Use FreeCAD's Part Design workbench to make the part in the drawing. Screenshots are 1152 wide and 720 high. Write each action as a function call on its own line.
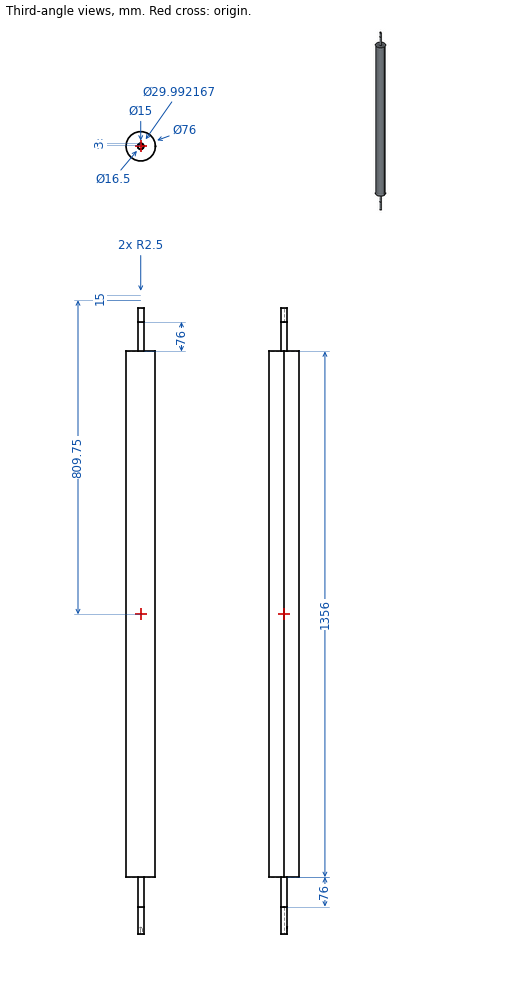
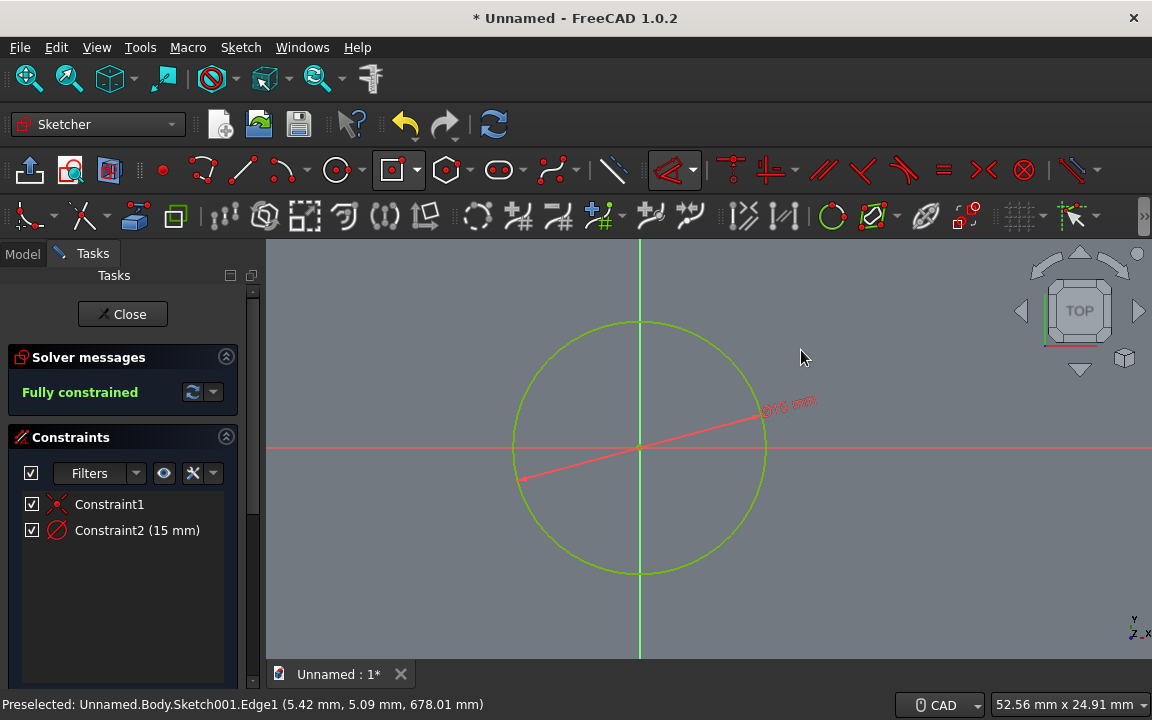
click(123, 314)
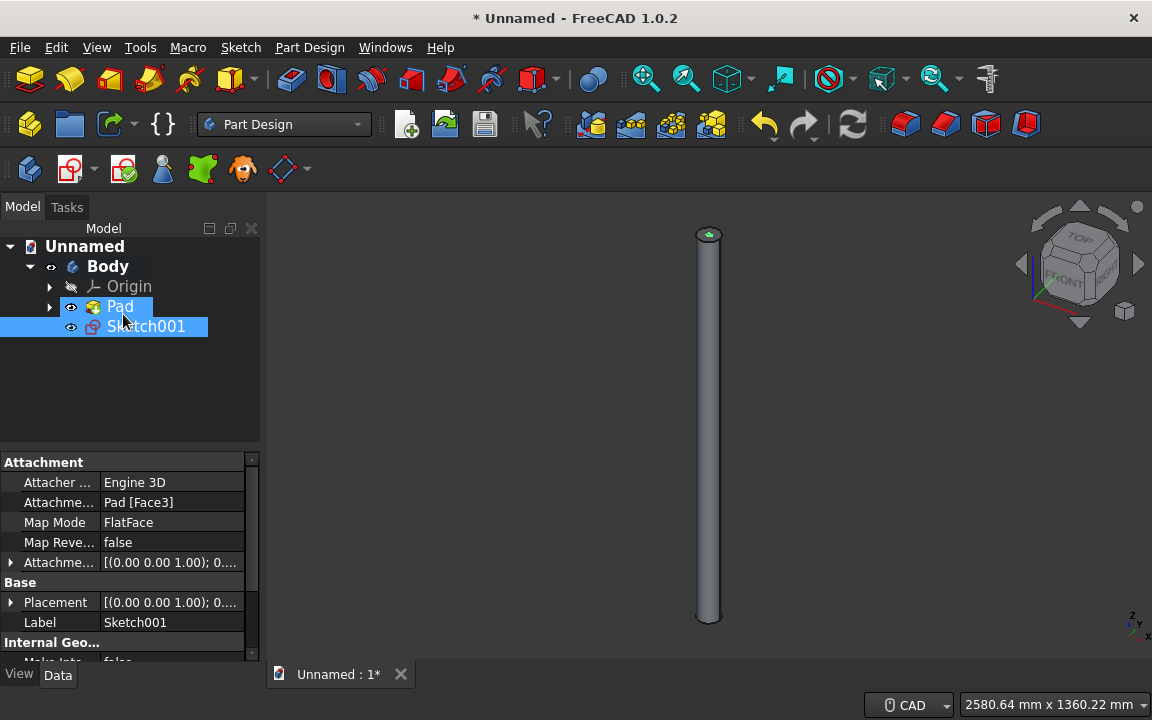
click(30, 80)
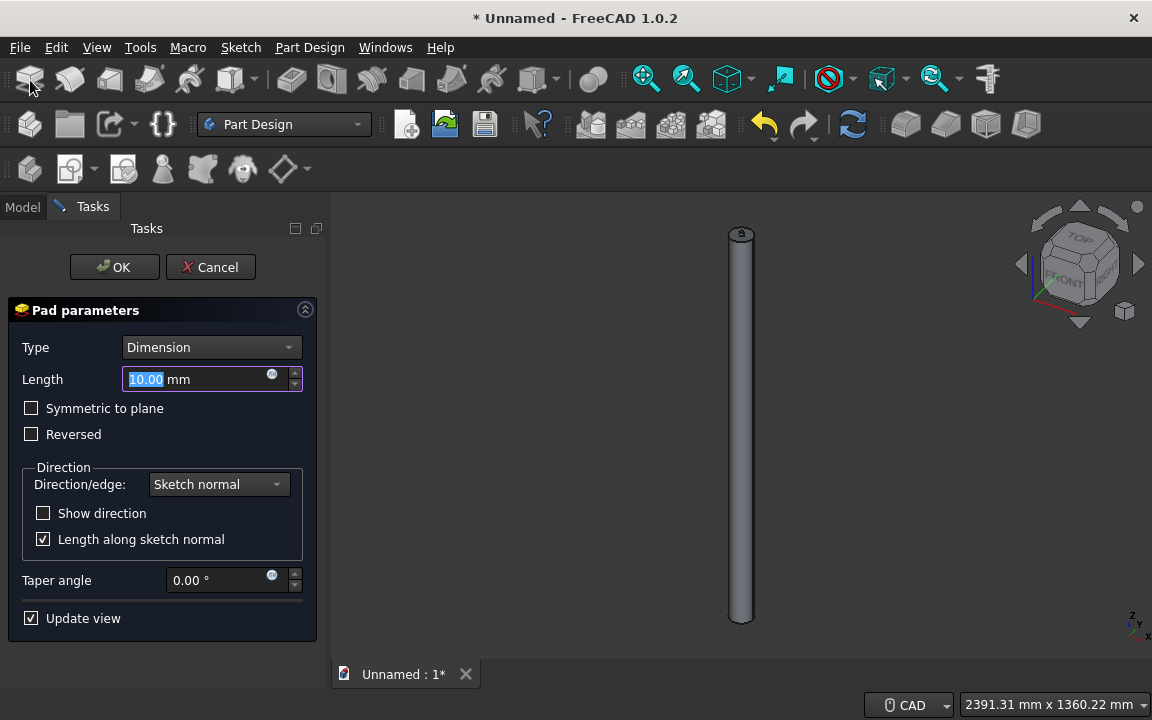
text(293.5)
key(Tab)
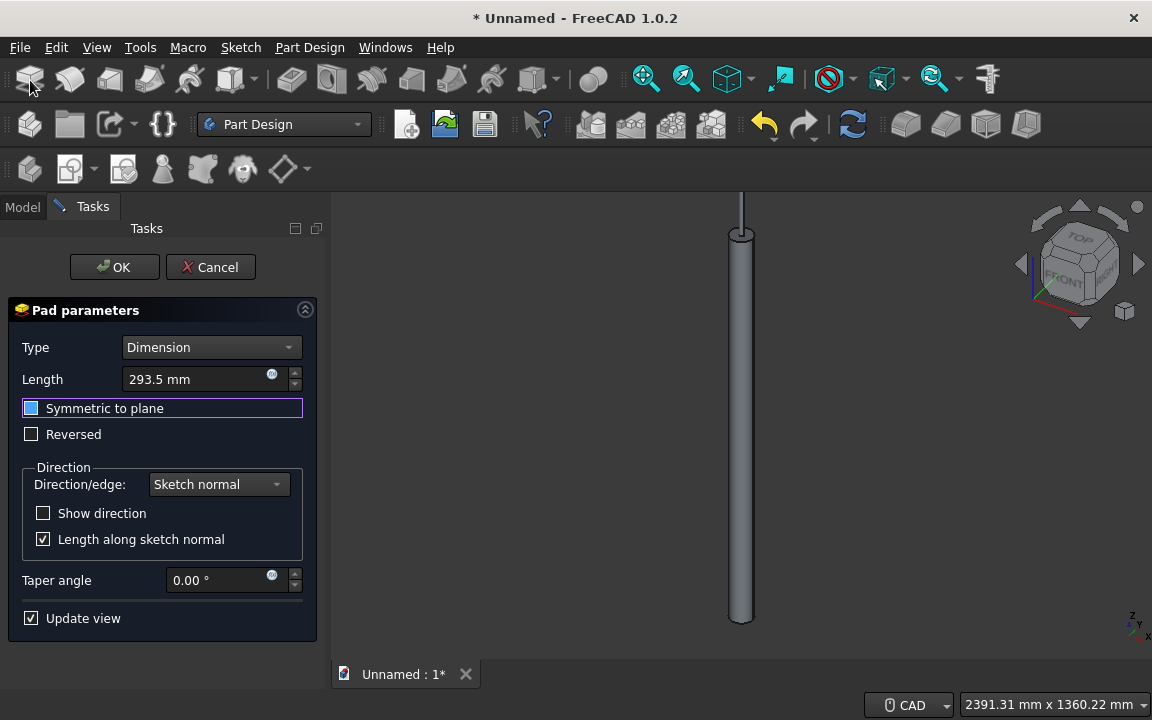
click(30, 408)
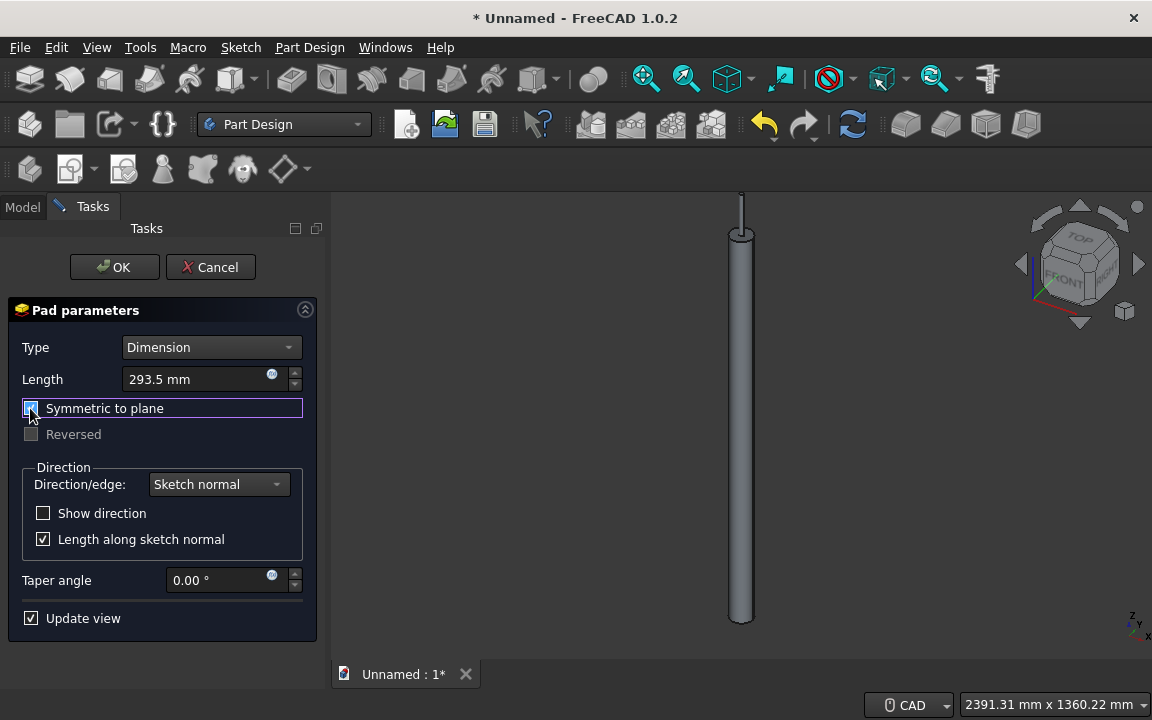
click(115, 267)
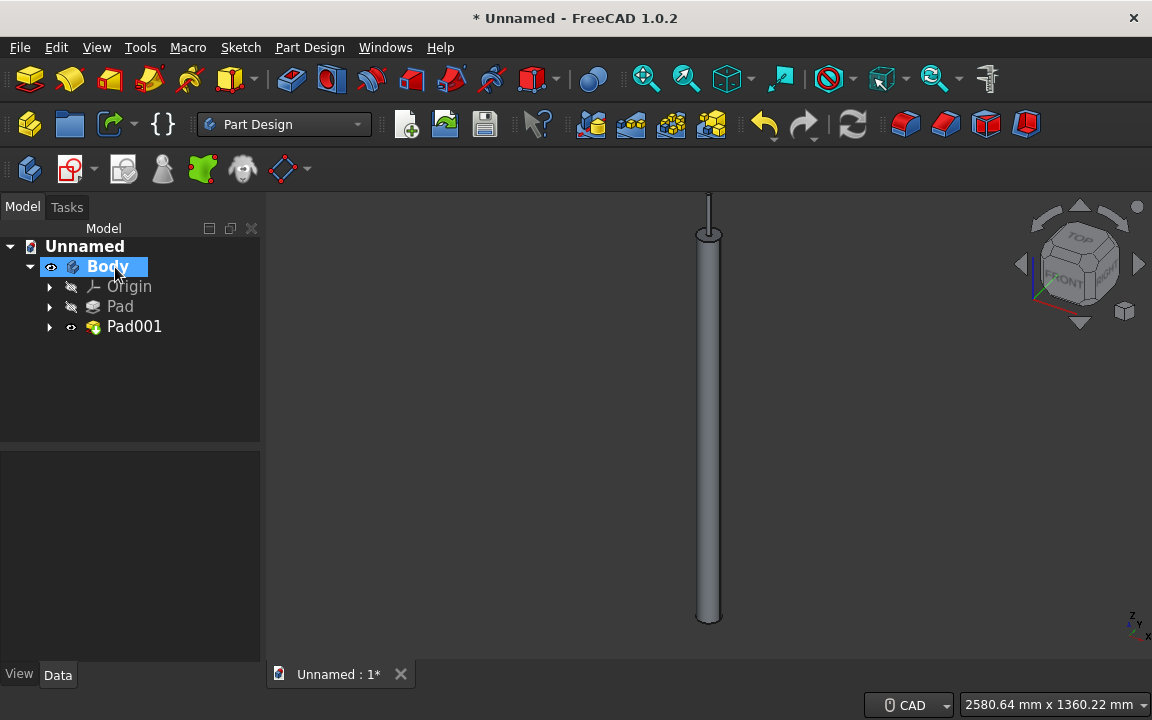
click(648, 80)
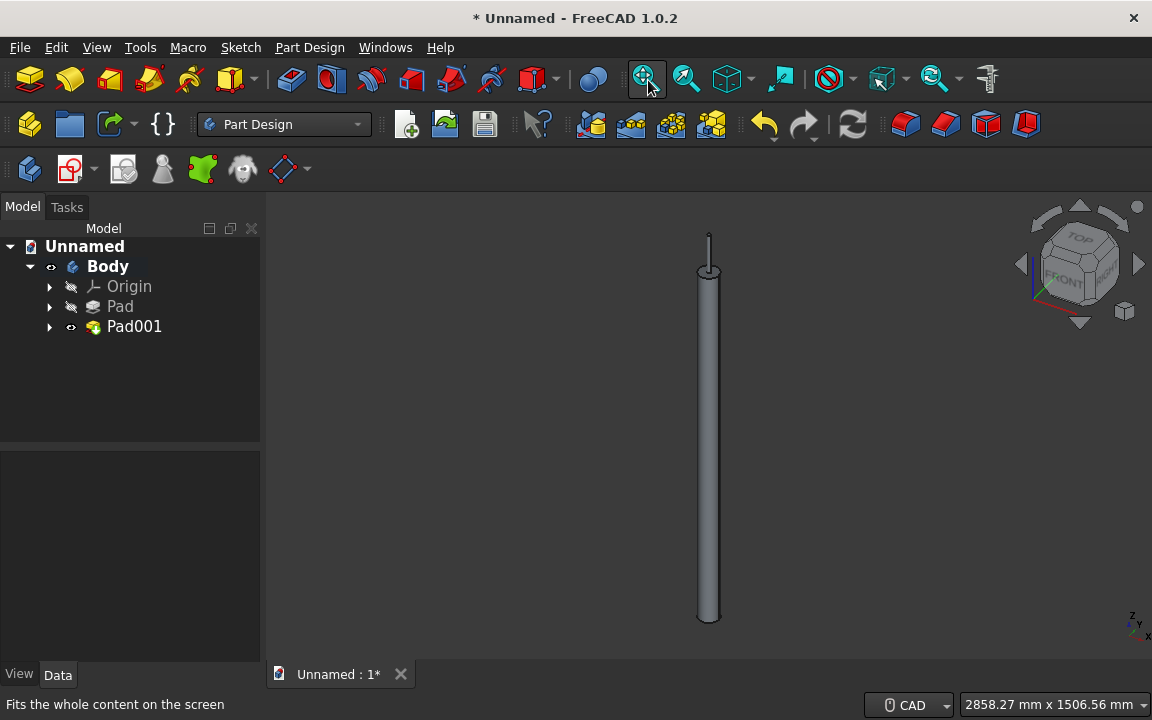
click(116, 327)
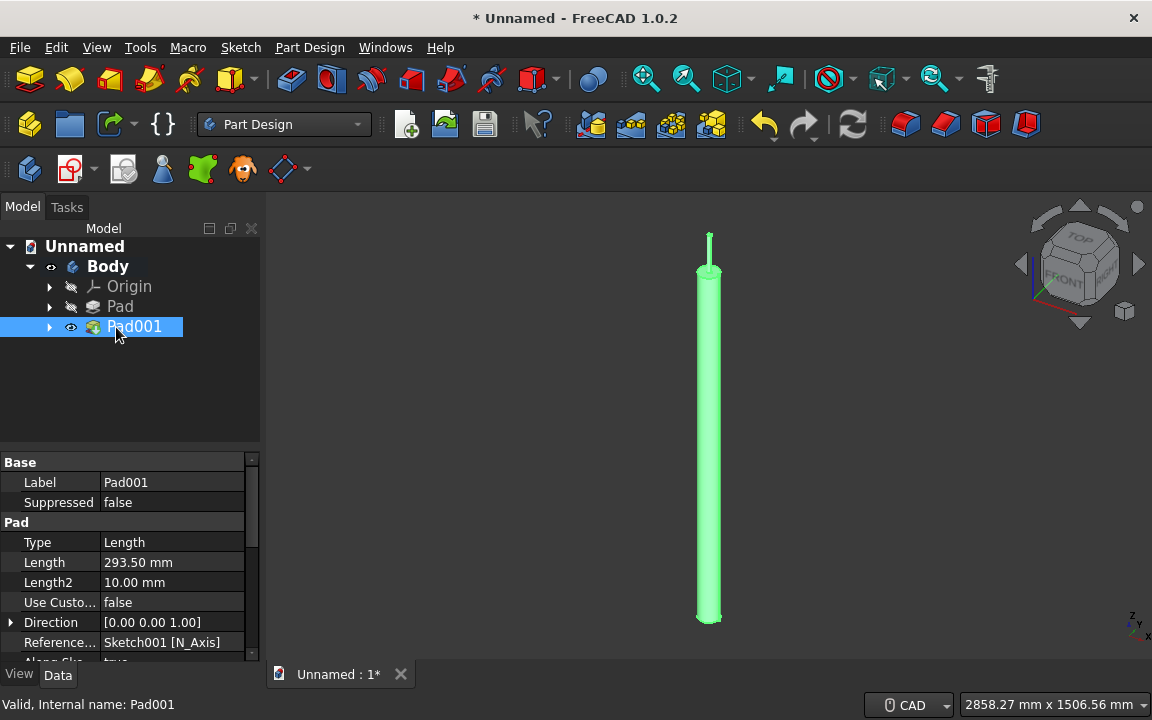
click(592, 124)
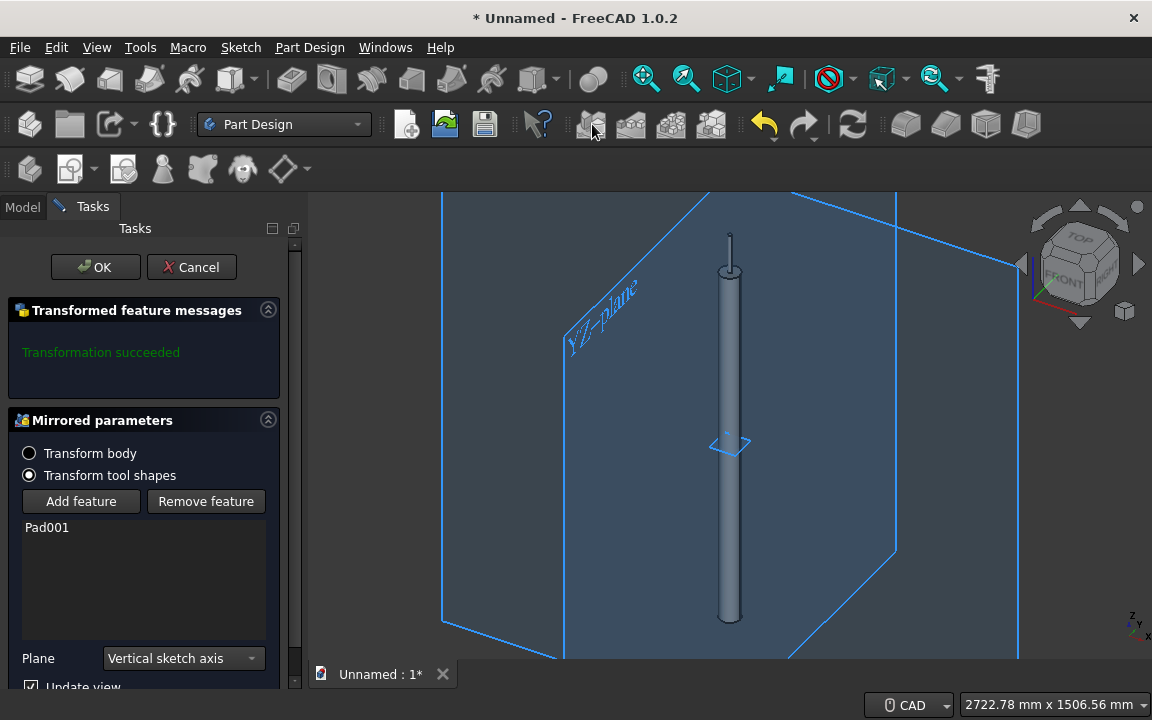
click(184, 658)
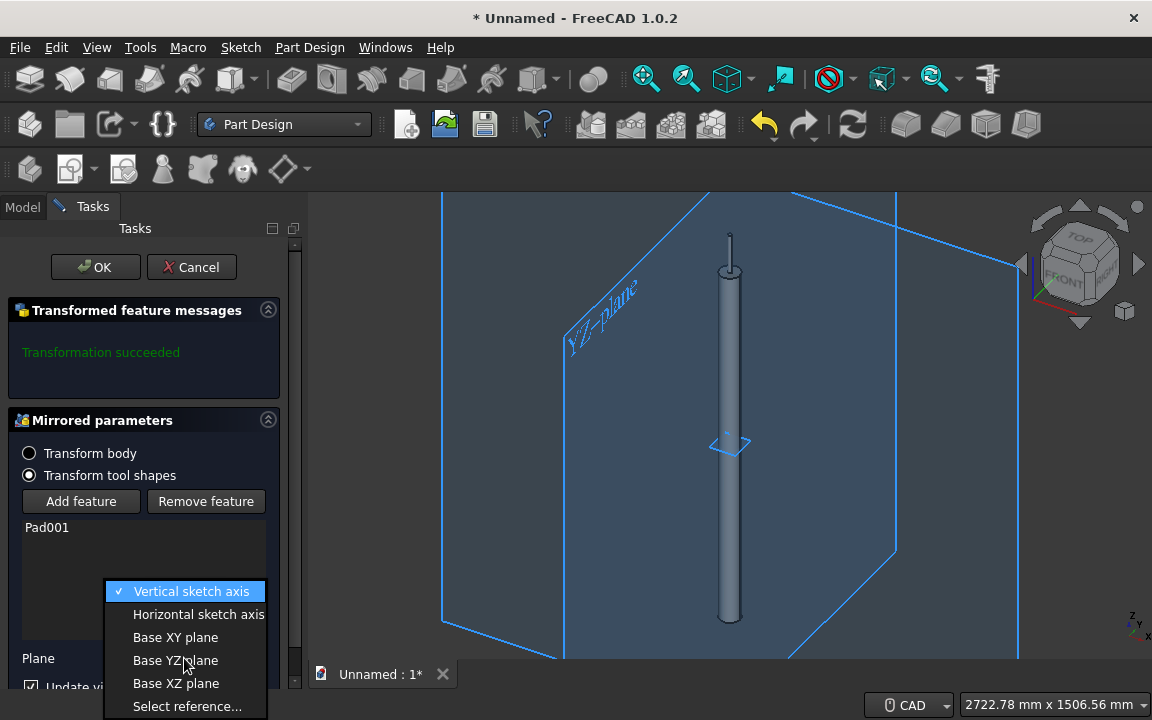
click(184, 638)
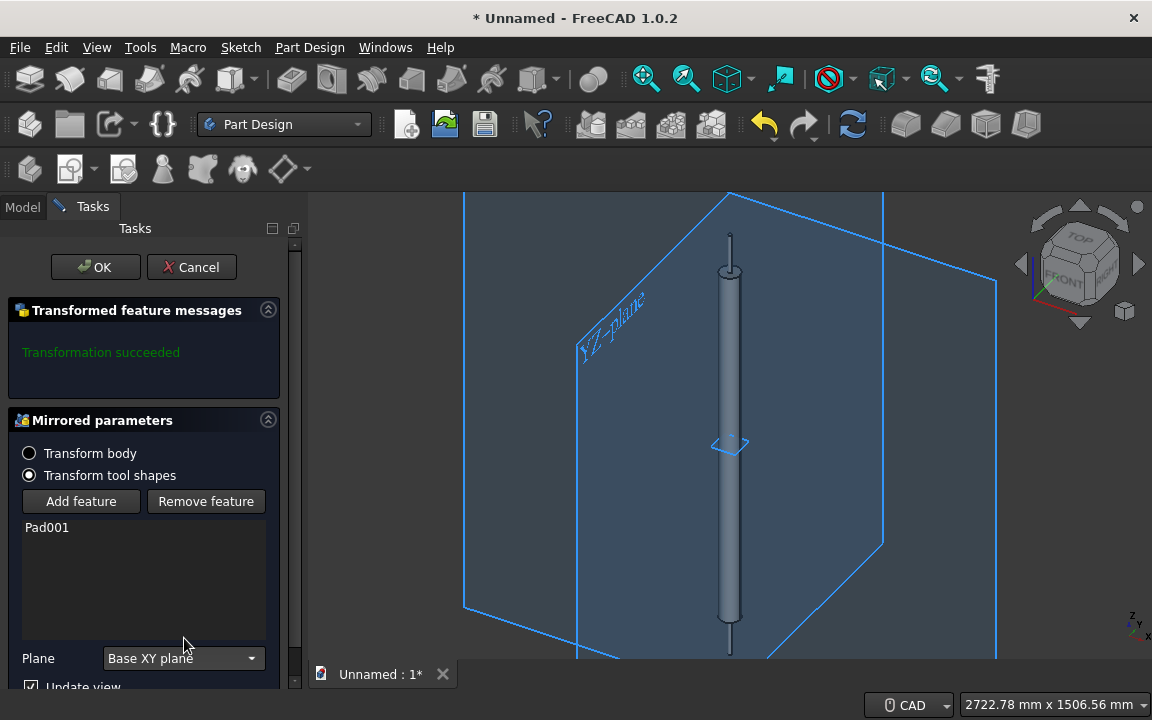
click(96, 267)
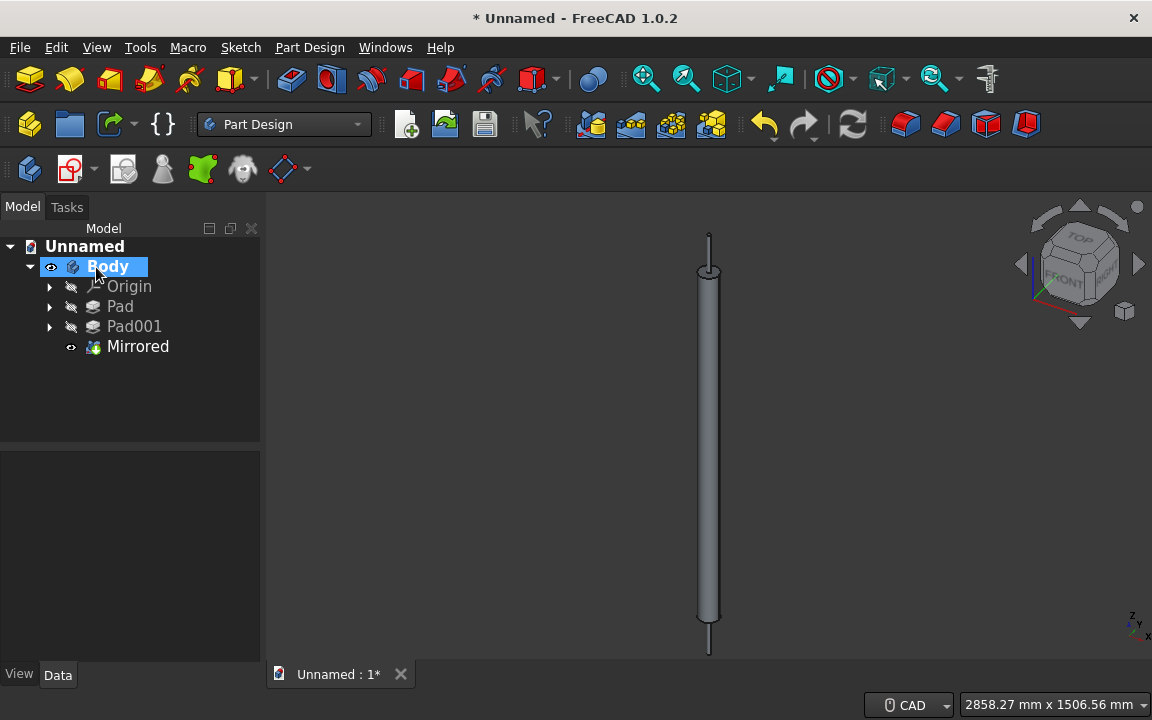
click(648, 80)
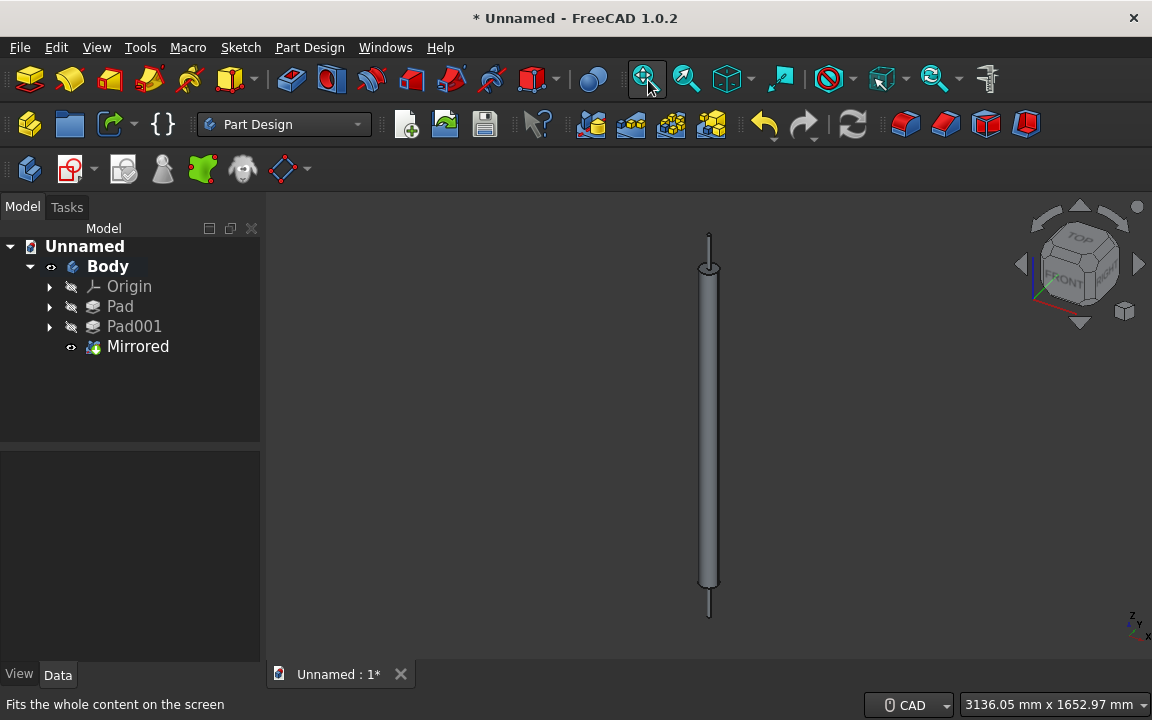
scroll(704, 266, up, 6)